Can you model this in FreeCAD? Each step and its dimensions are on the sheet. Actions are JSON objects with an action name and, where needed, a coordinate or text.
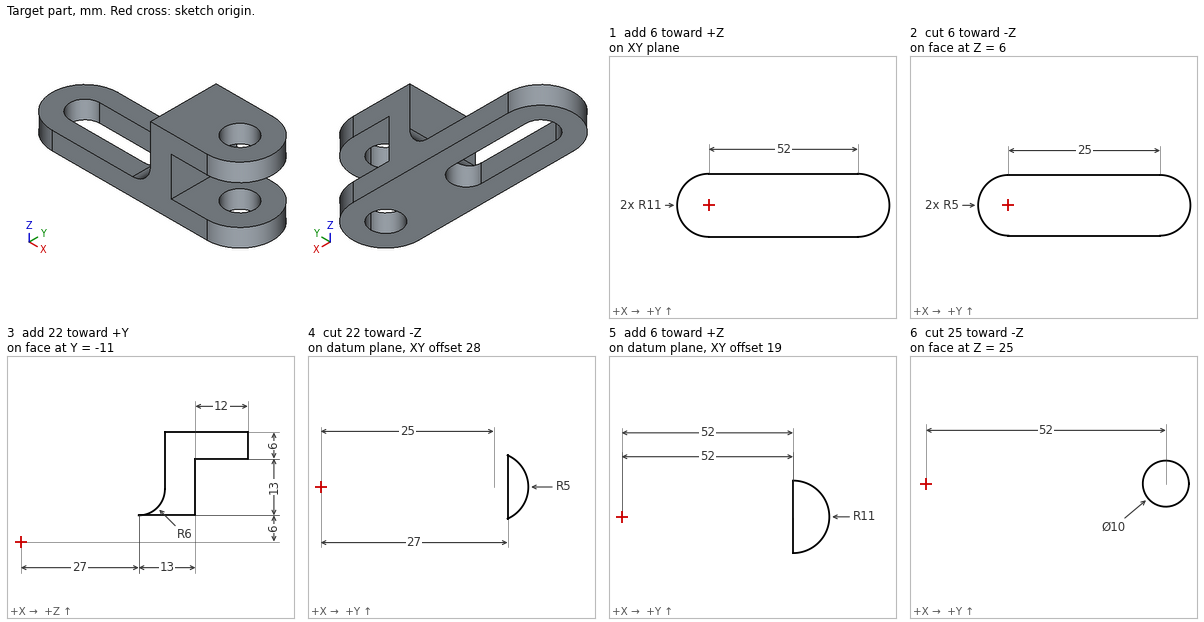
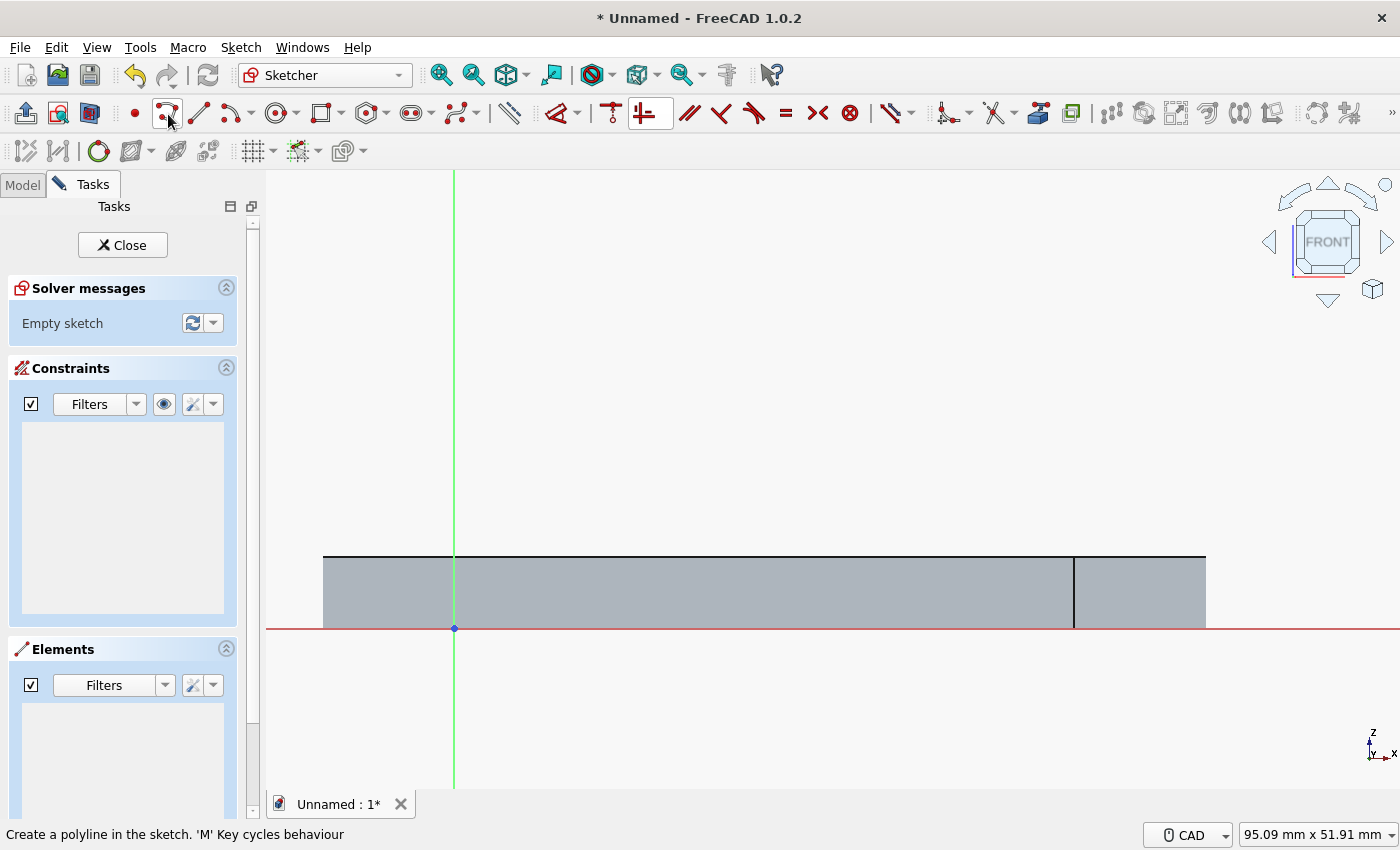
{"action": "left_click", "coordinate": [776, 557]}
{"action": "left_click", "coordinate": [931, 557]}
{"action": "left_click", "coordinate": [931, 402]}
{"action": "left_click", "coordinate": [1074, 402]}
{"action": "left_click", "coordinate": [1074, 330]}
{"action": "left_click", "coordinate": [848, 330]}
{"action": "left_click", "coordinate": [848, 485]}
{"action": "right_click", "coordinate": [848, 485]}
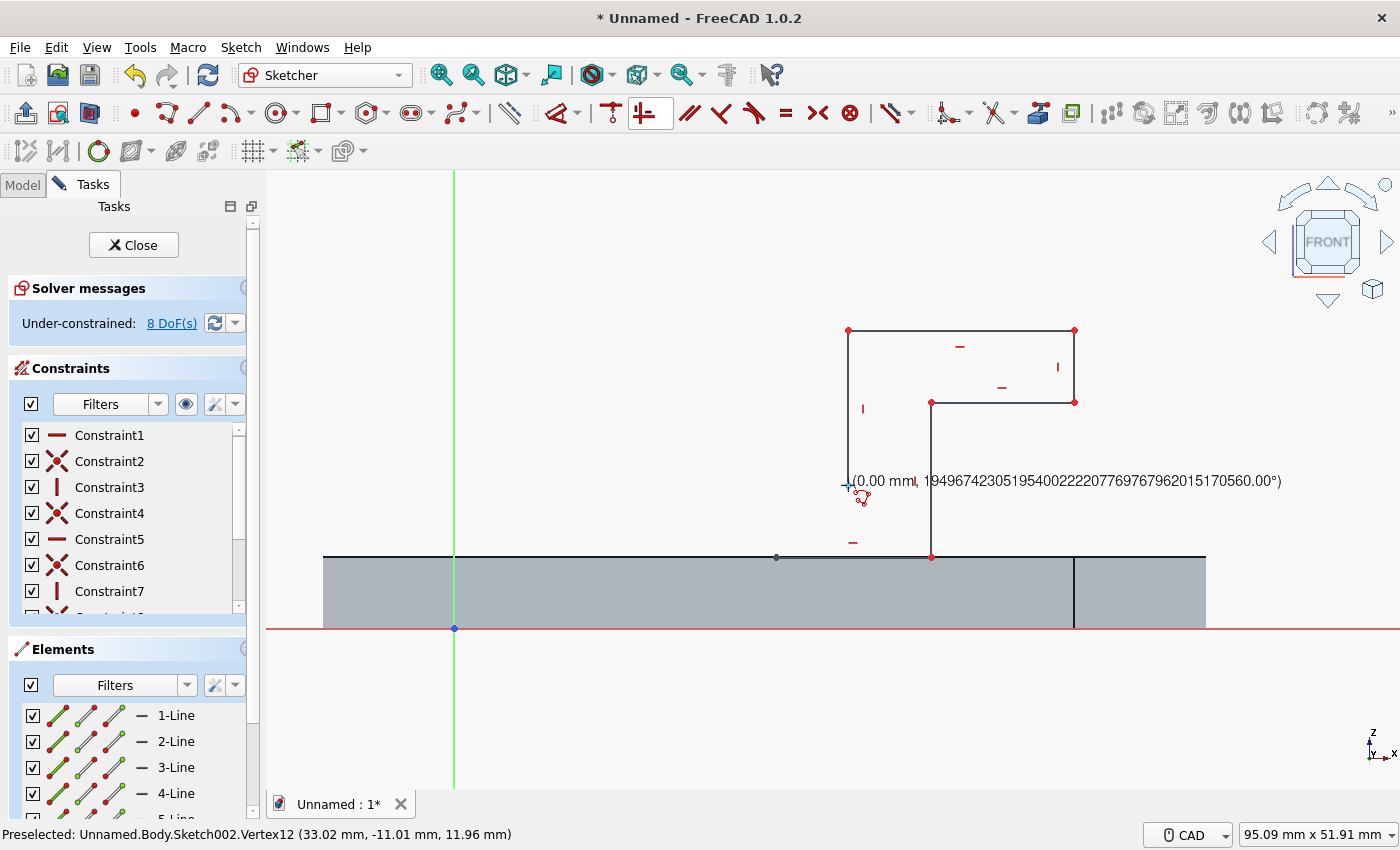
{"action": "left_click", "coordinate": [254, 114]}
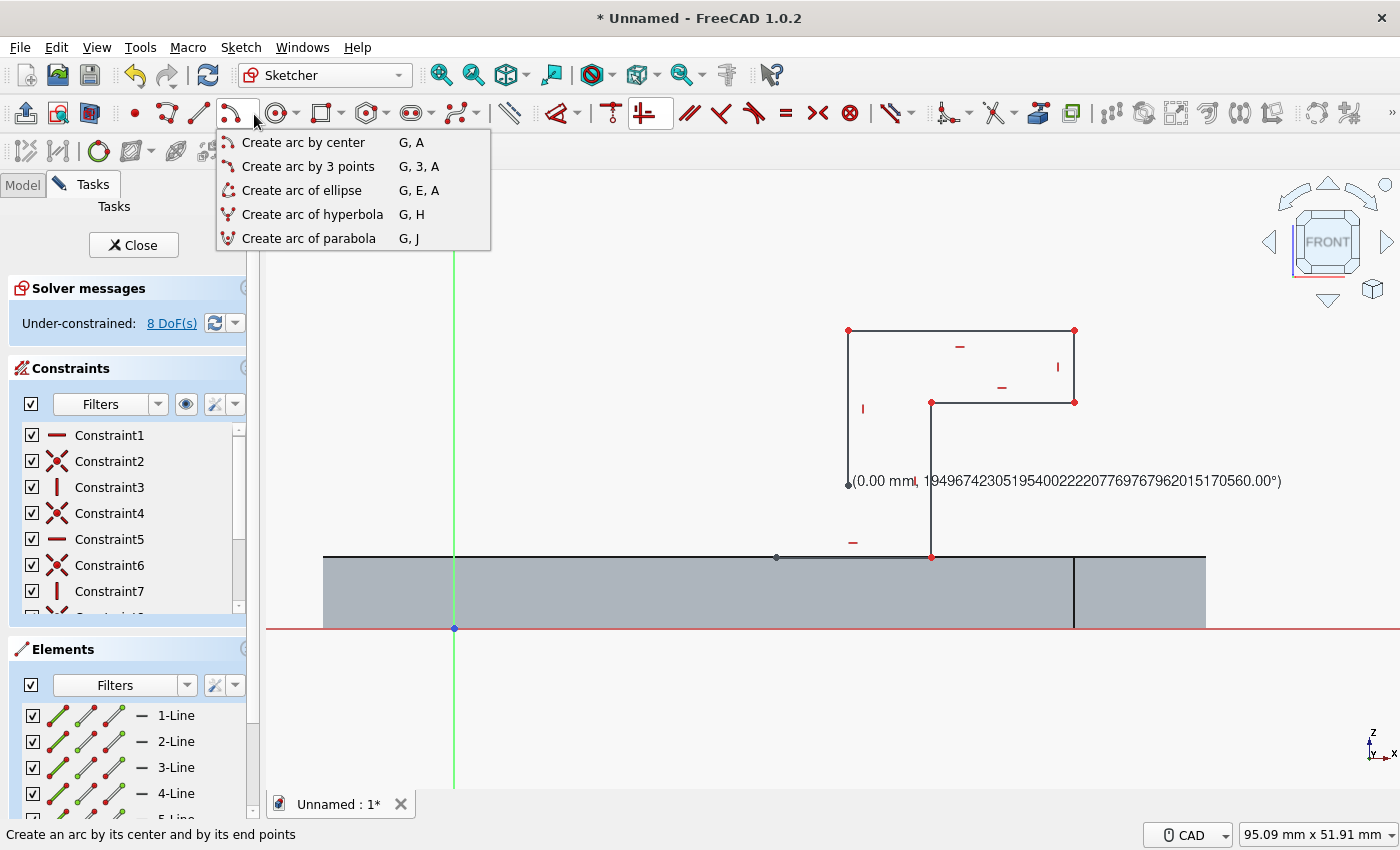
{"action": "left_click", "coordinate": [354, 166]}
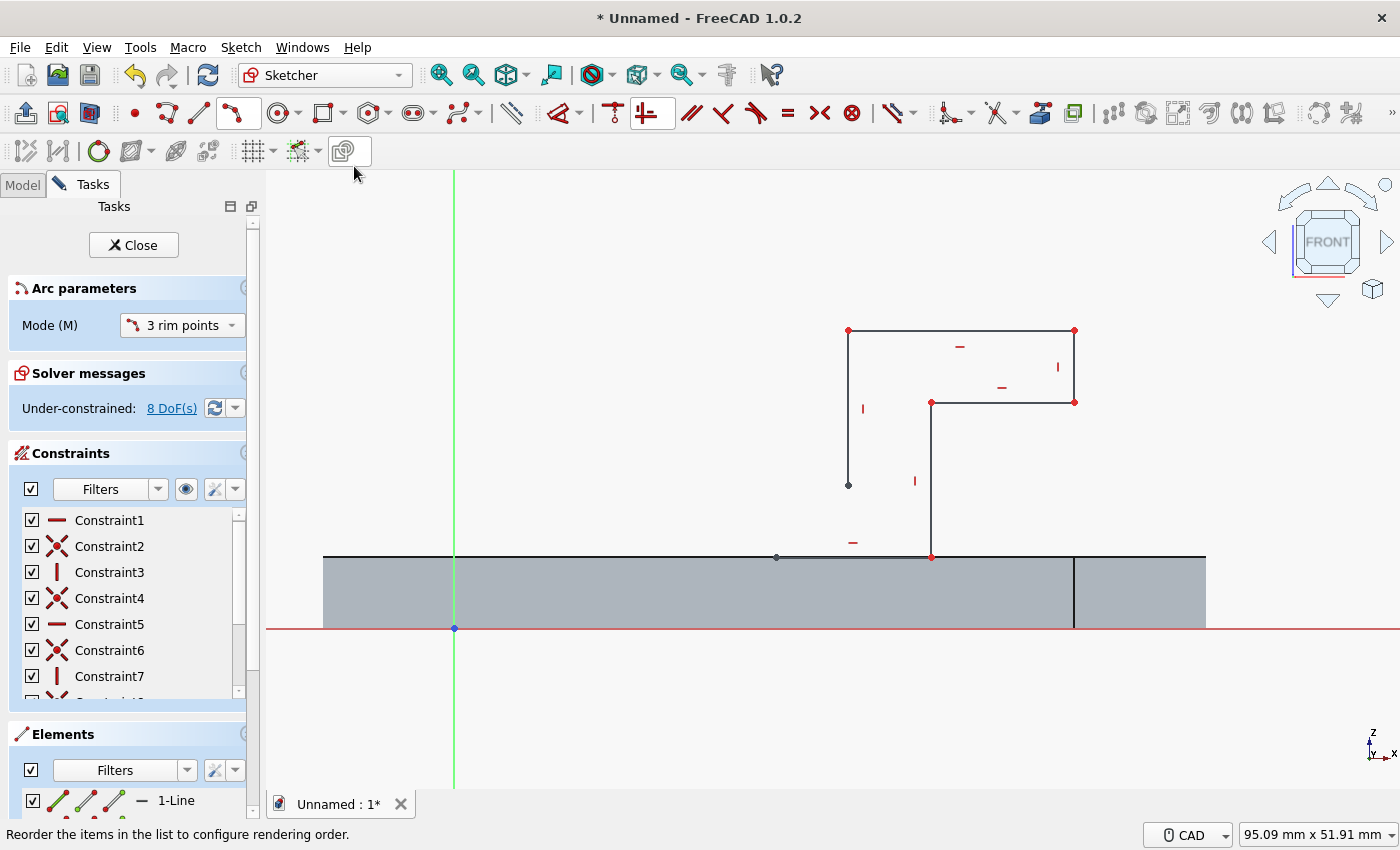
{"action": "left_click", "coordinate": [848, 486]}
{"action": "left_click", "coordinate": [776, 558]}
{"action": "left_click", "coordinate": [827, 536]}
{"action": "key", "text": "Escape"}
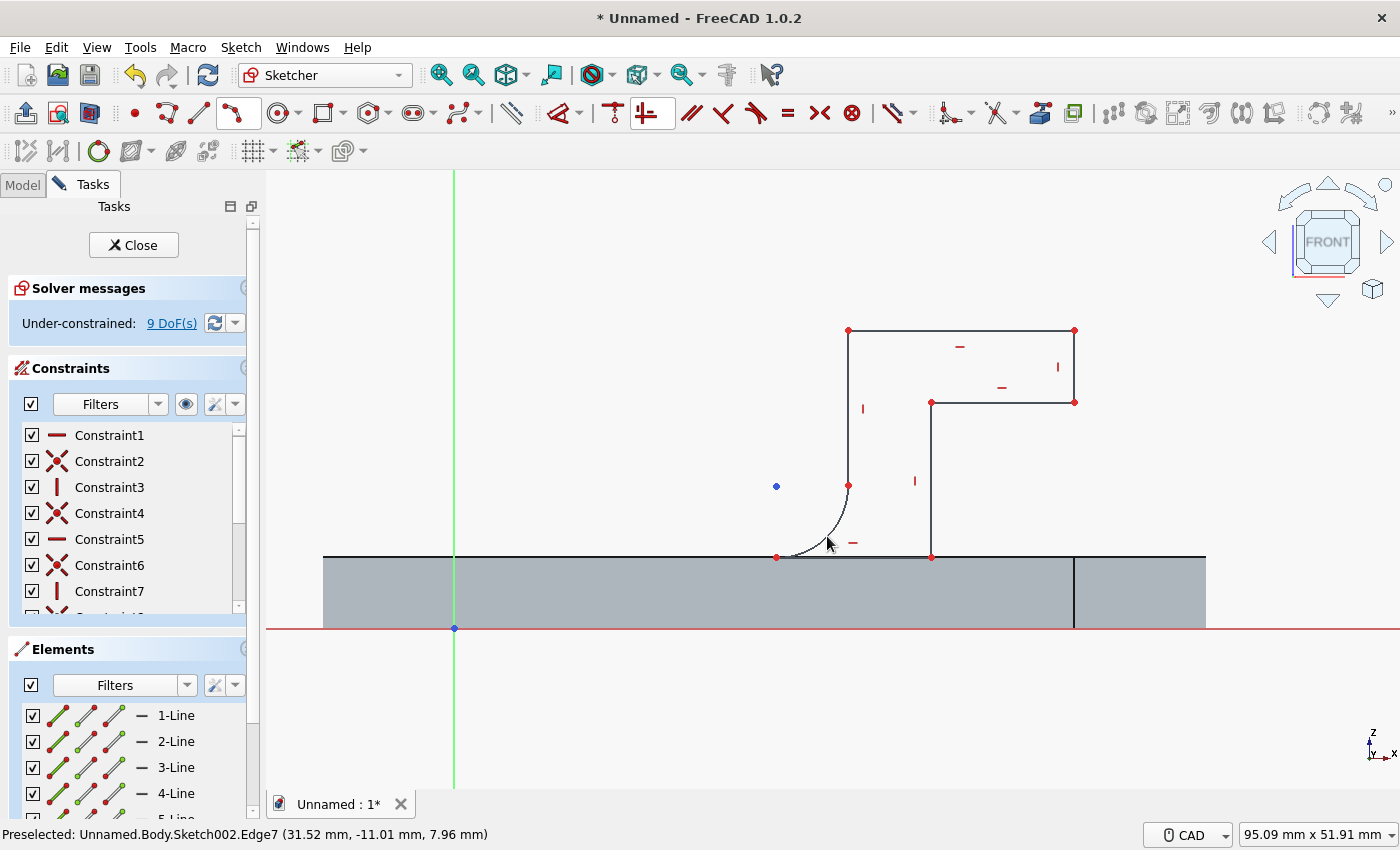
{"action": "left_click", "coordinate": [823, 558]}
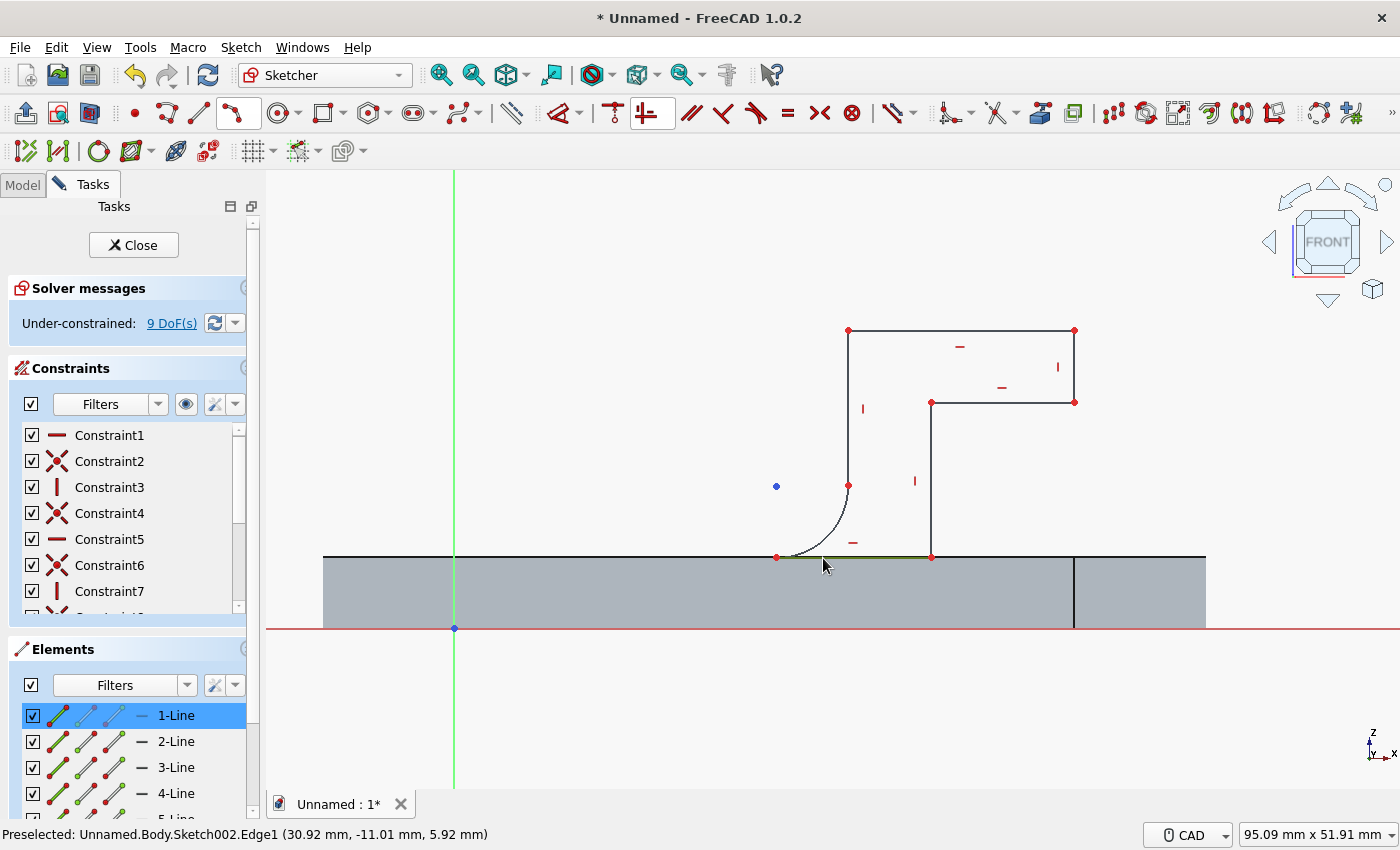
{"action": "left_click", "coordinate": [840, 519]}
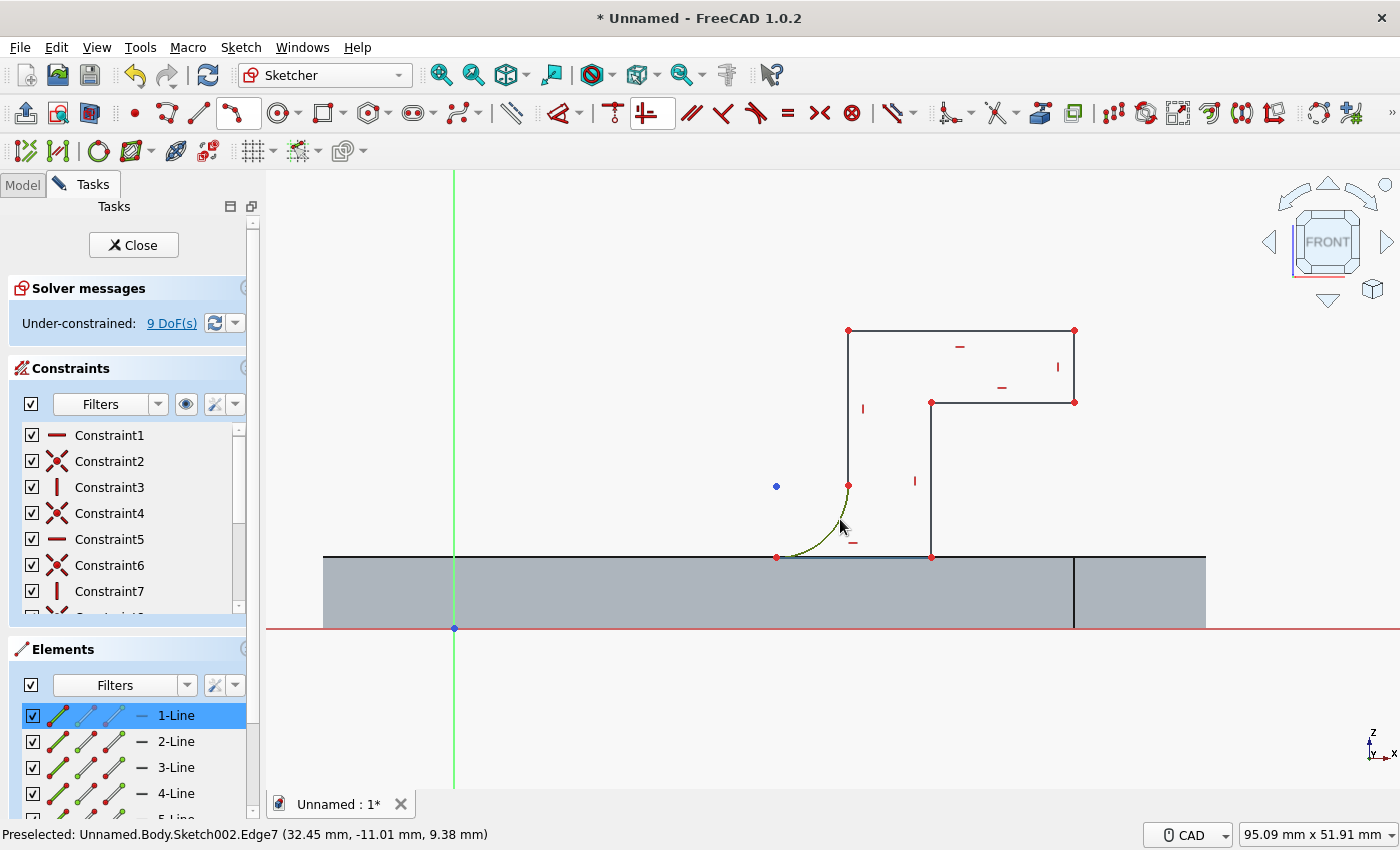
{"action": "left_click", "coordinate": [756, 114]}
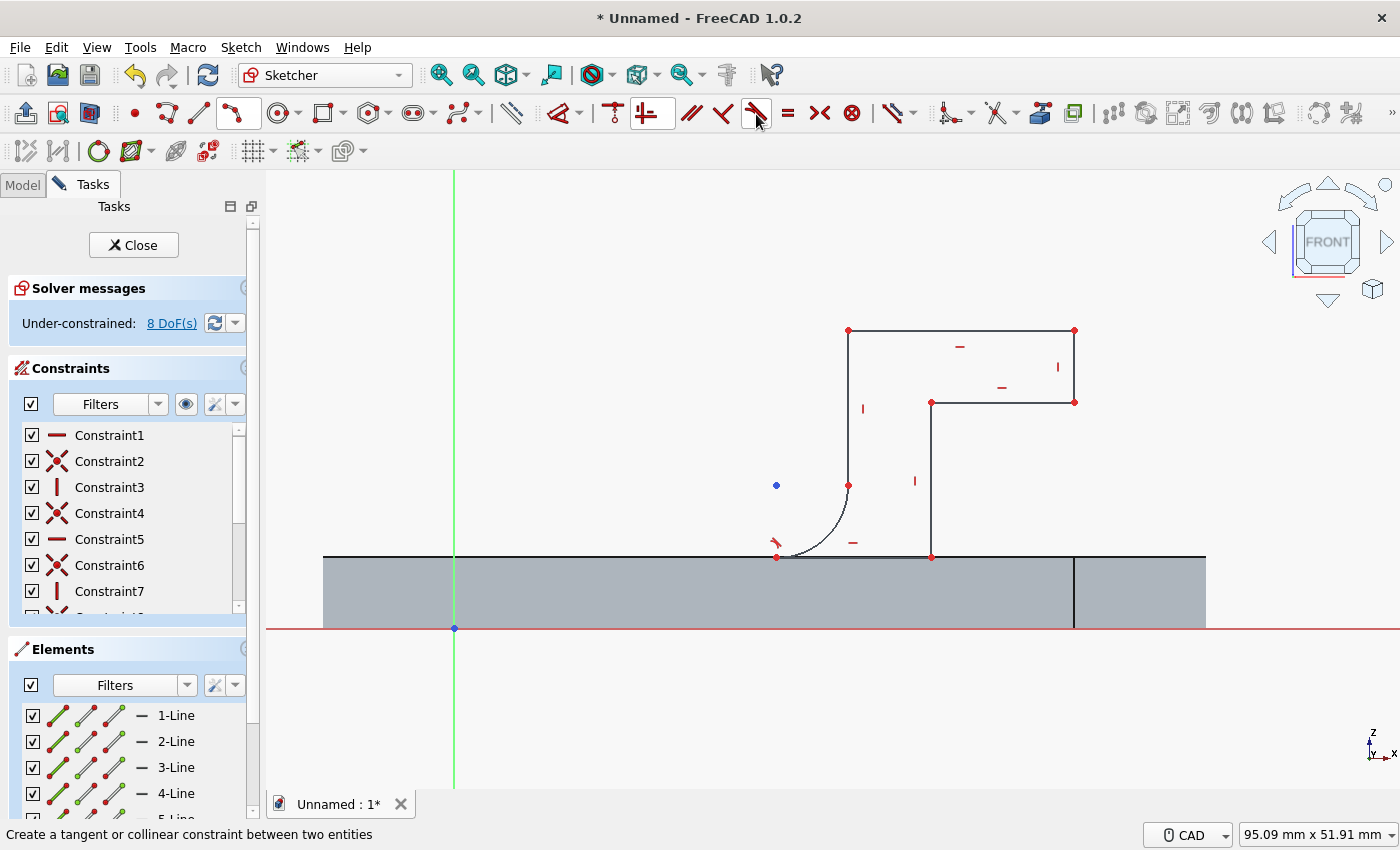
{"action": "left_click", "coordinate": [848, 377]}